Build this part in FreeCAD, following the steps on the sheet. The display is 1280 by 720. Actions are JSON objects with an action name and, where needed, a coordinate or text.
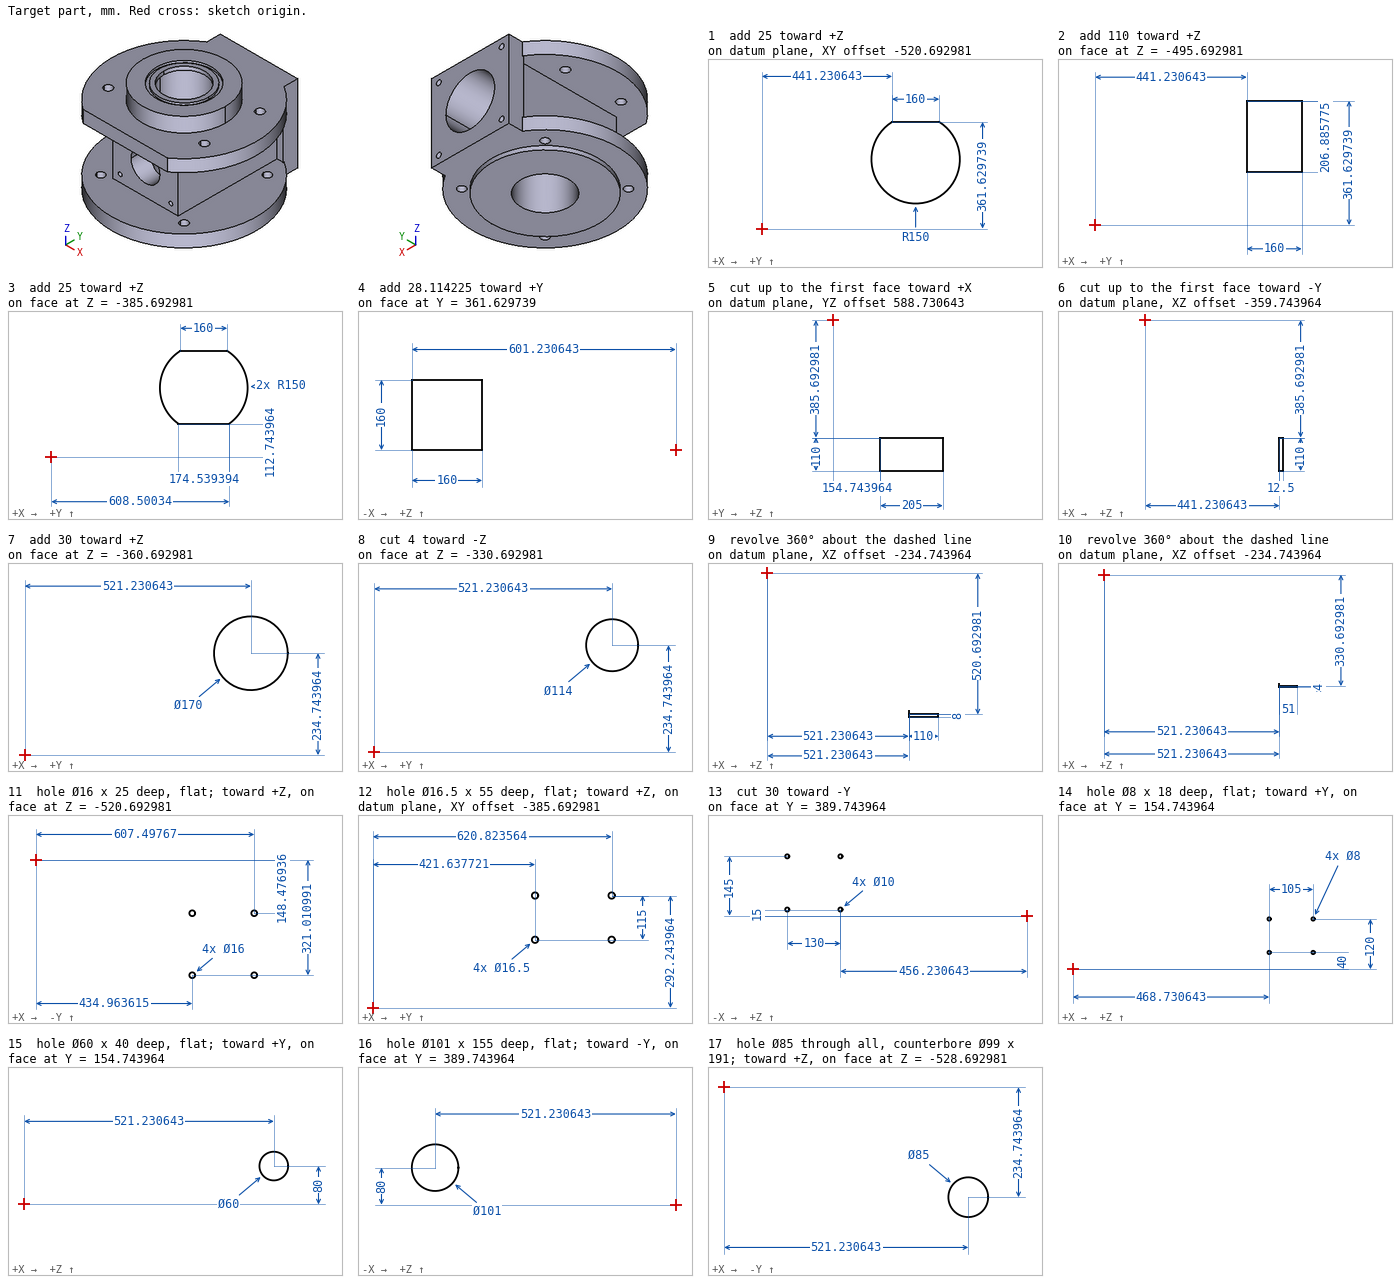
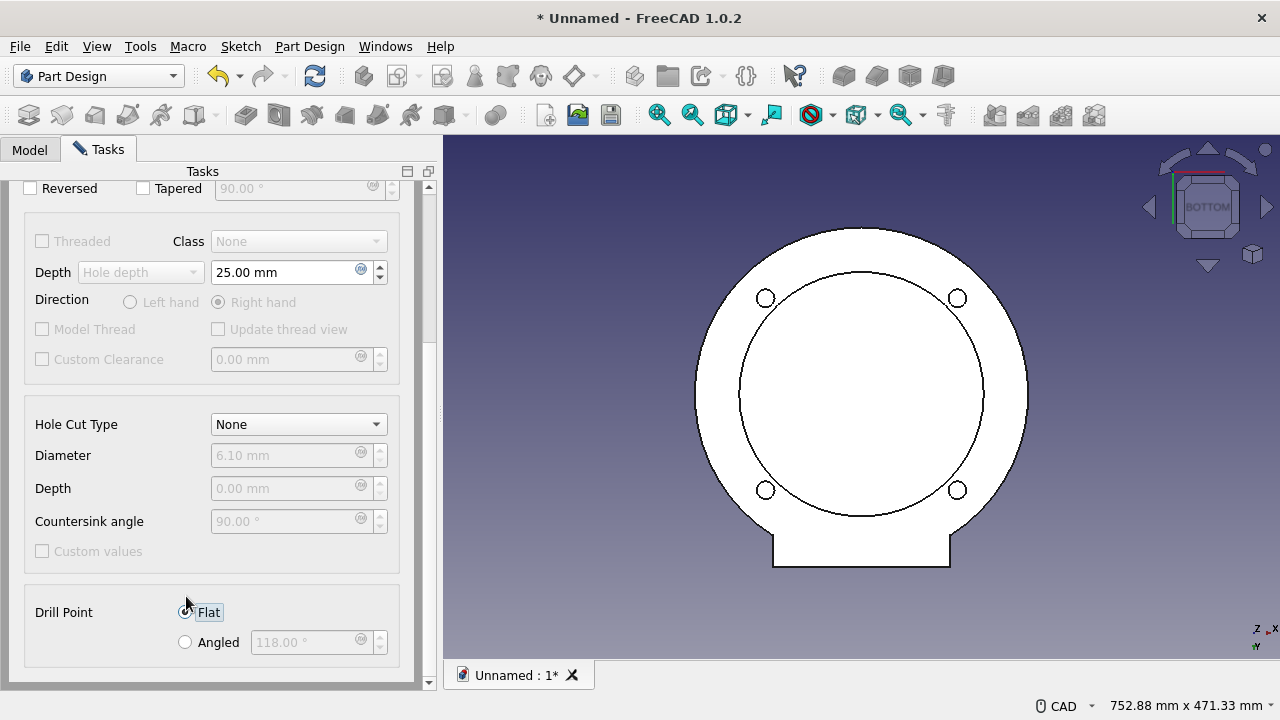
{"action": "scroll", "coordinate": [429, 436], "scroll_direction": "up", "scroll_amount": 5}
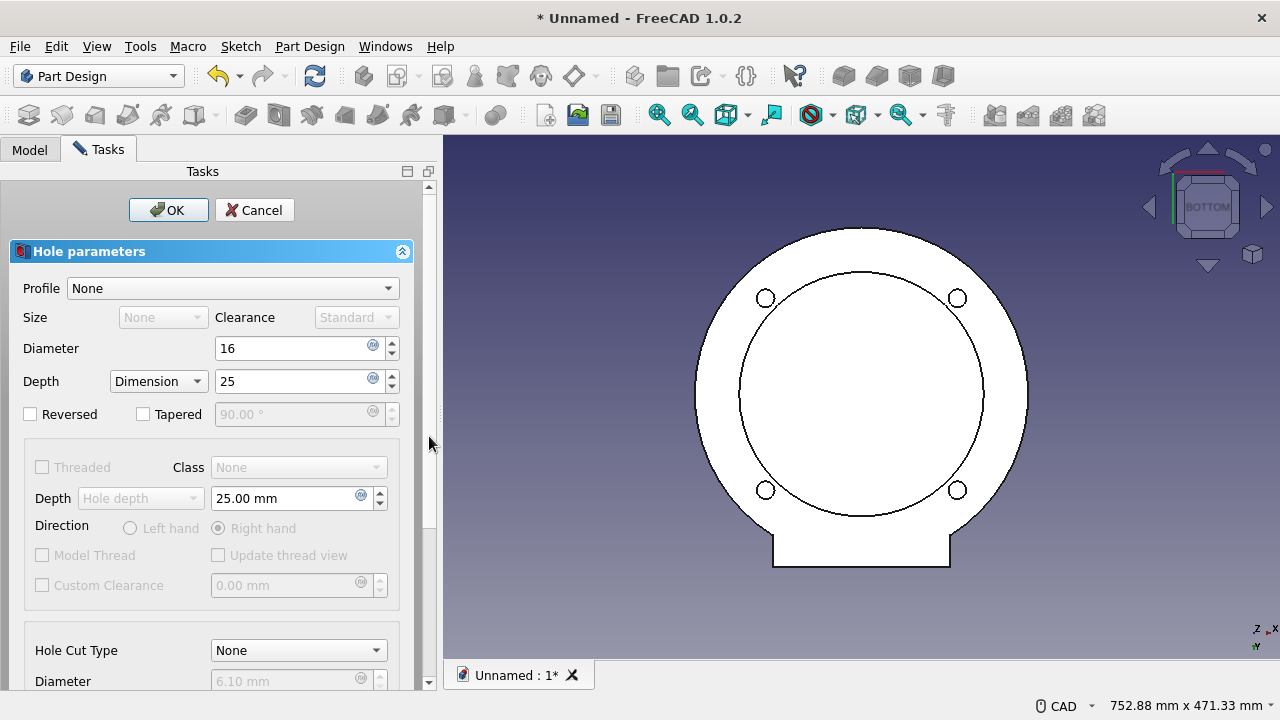
{"action": "left_click", "coordinate": [169, 210]}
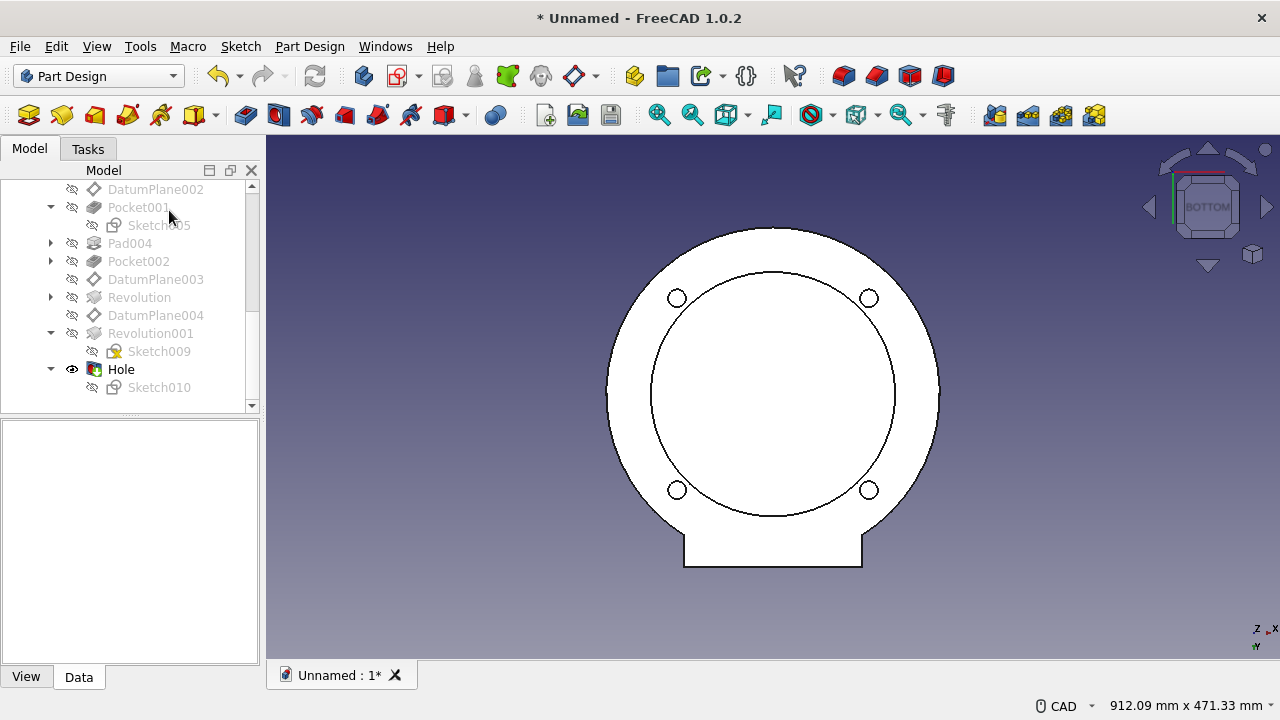
{"action": "scroll", "coordinate": [141, 293], "scroll_direction": "down", "scroll_amount": 3}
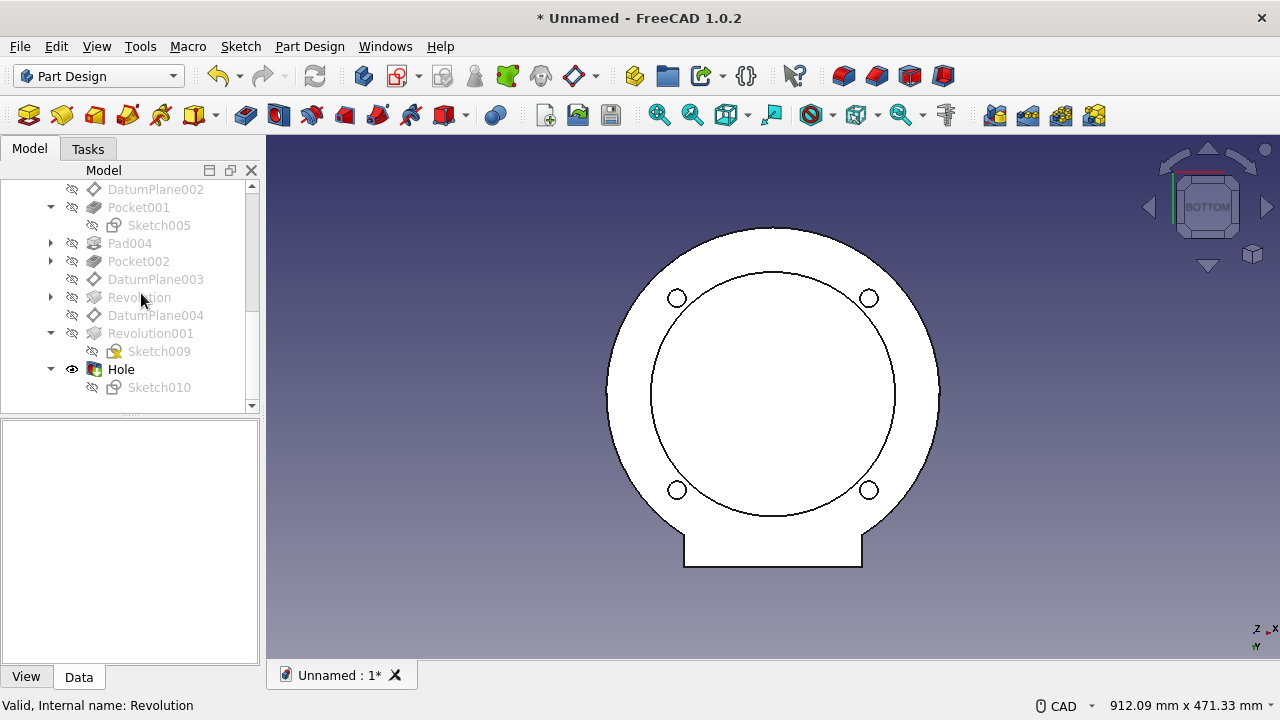
{"action": "scroll", "coordinate": [141, 293], "scroll_direction": "up", "scroll_amount": 15}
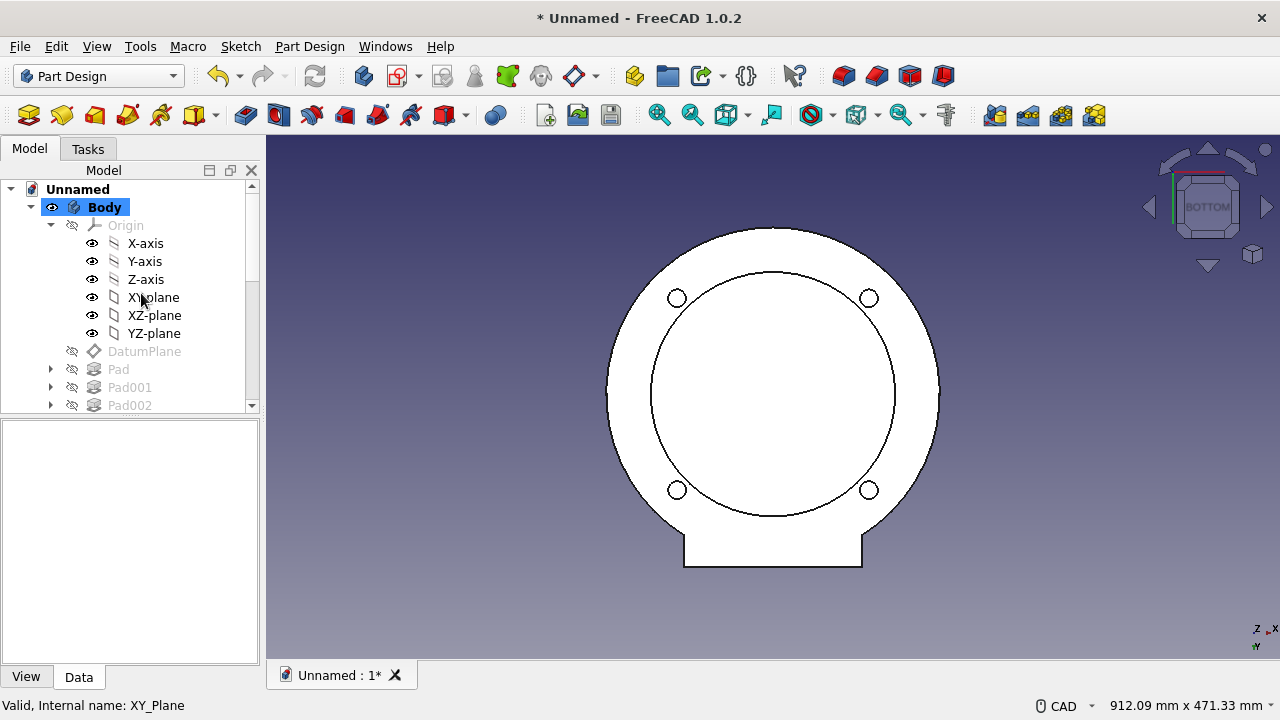
{"action": "left_click", "coordinate": [137, 297]}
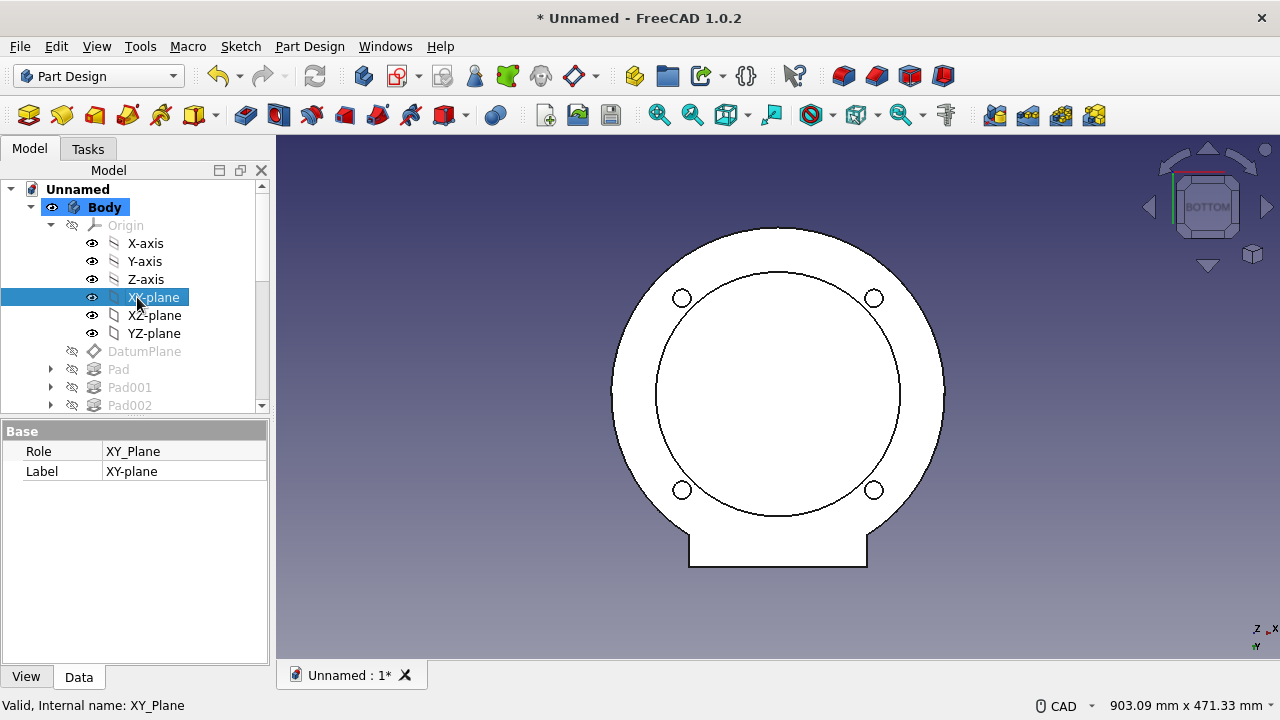
{"action": "left_click", "coordinate": [574, 76]}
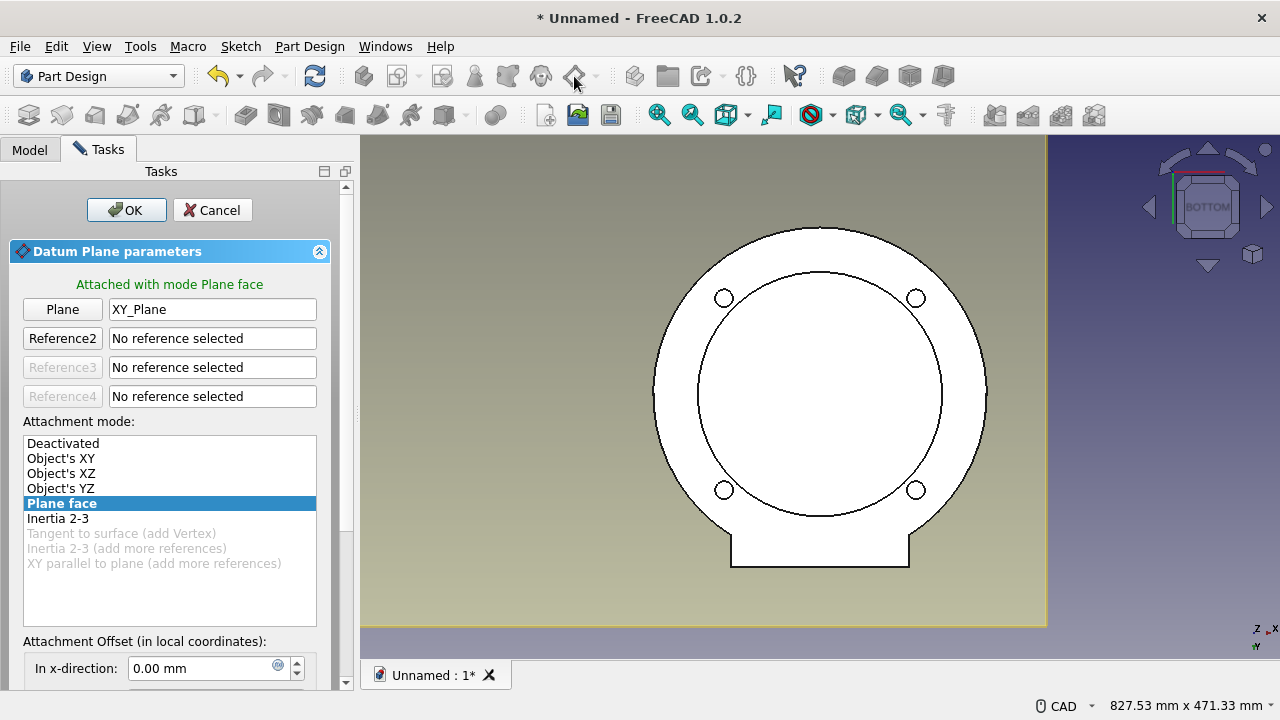
{"action": "scroll", "coordinate": [346, 436], "scroll_direction": "down", "scroll_amount": 2}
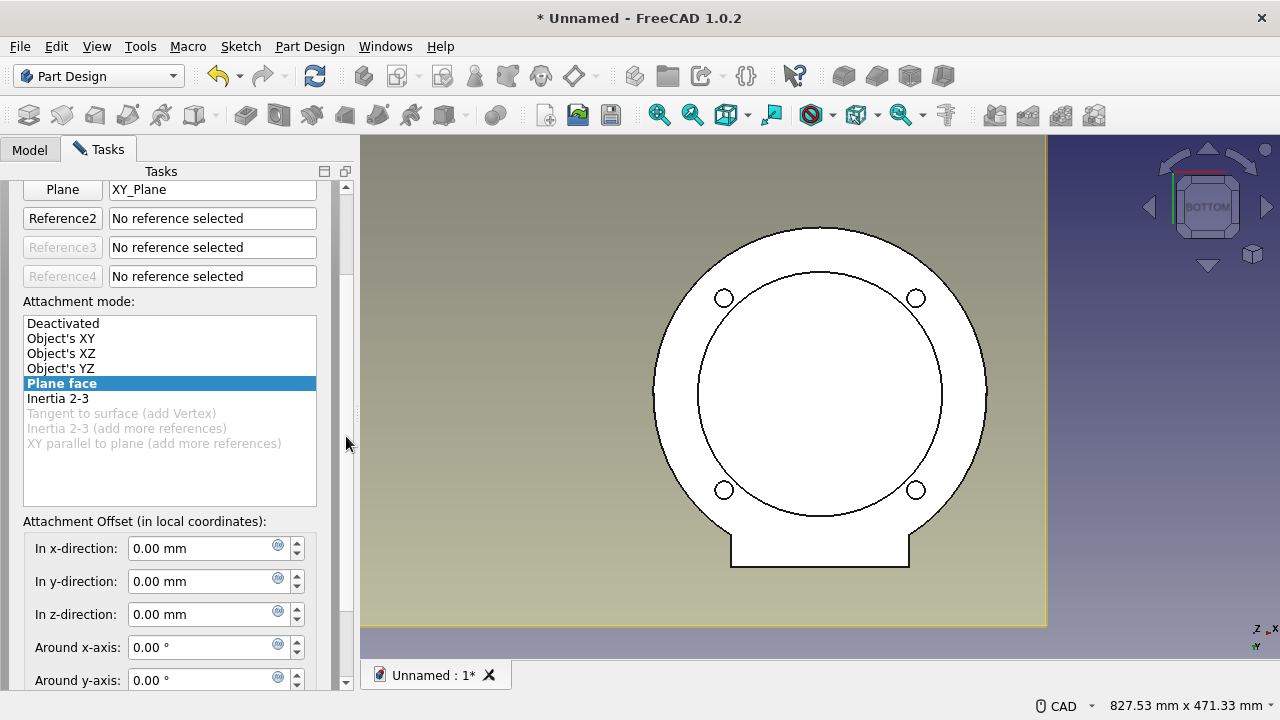
{"action": "triple_click", "coordinate": [210, 614]}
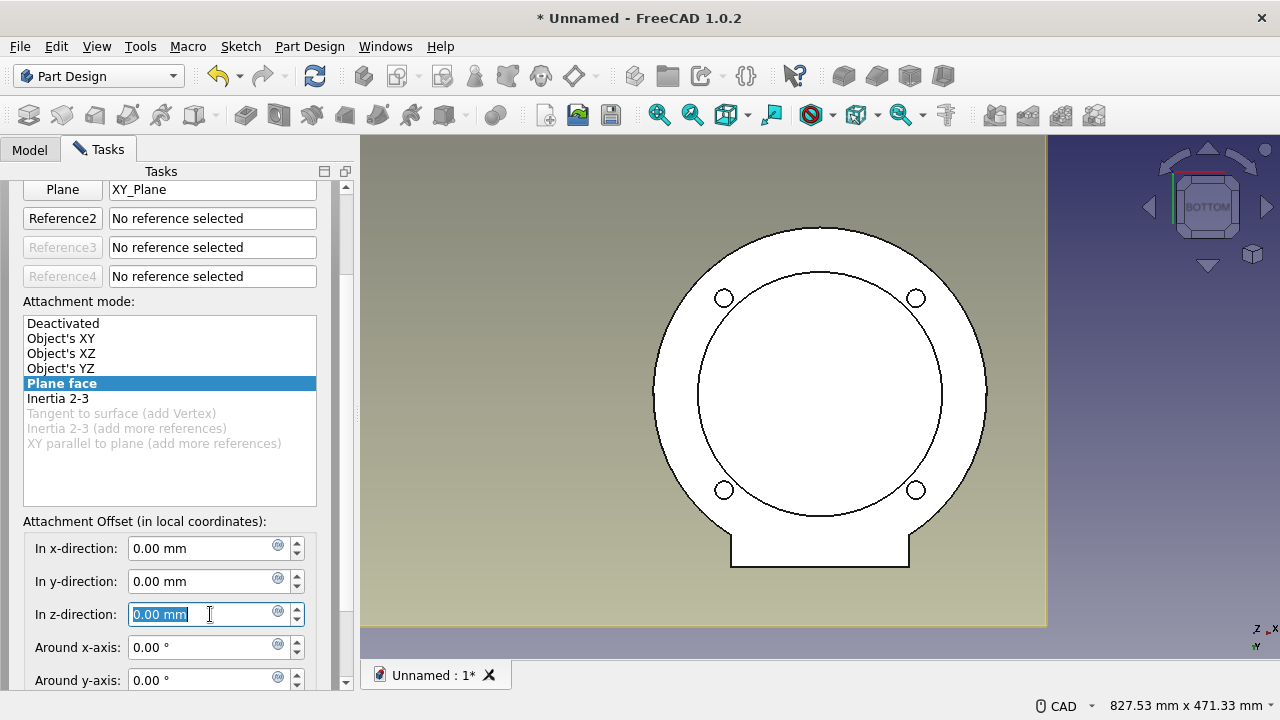
{"action": "type", "text": "-385.692981"}
{"action": "key", "text": "Tab"}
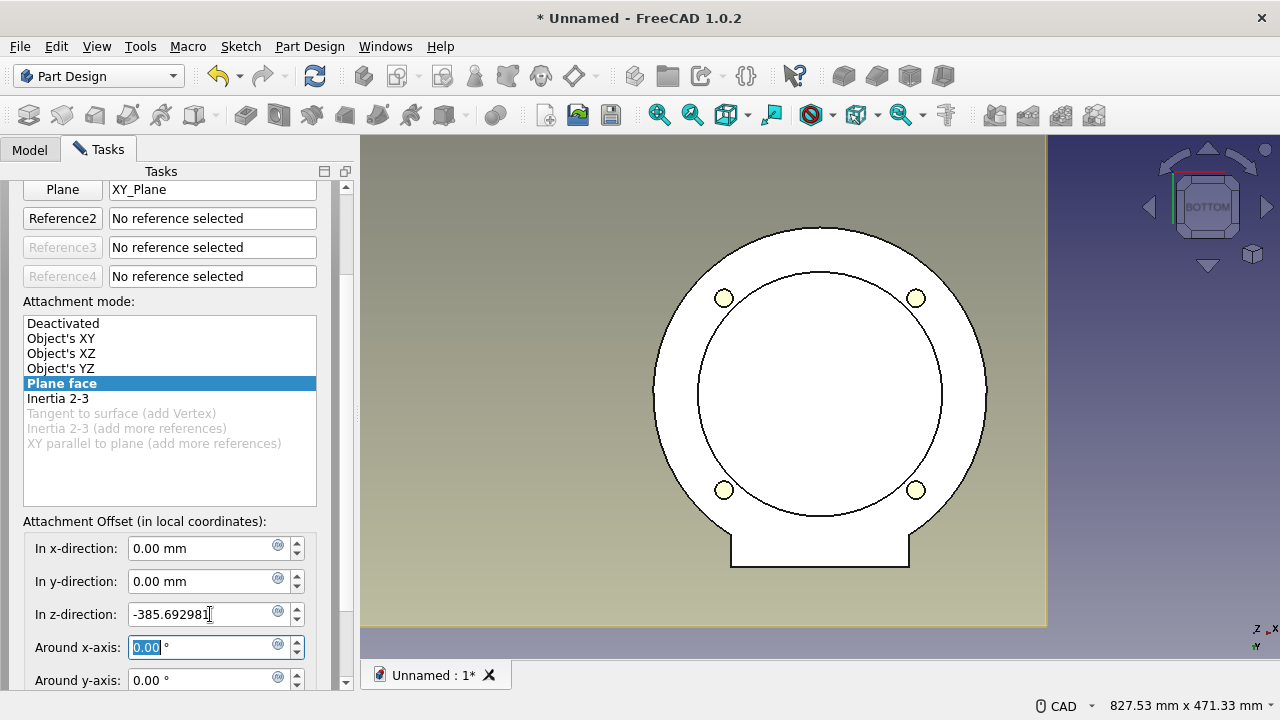
{"action": "scroll", "coordinate": [346, 436], "scroll_direction": "up", "scroll_amount": 3}